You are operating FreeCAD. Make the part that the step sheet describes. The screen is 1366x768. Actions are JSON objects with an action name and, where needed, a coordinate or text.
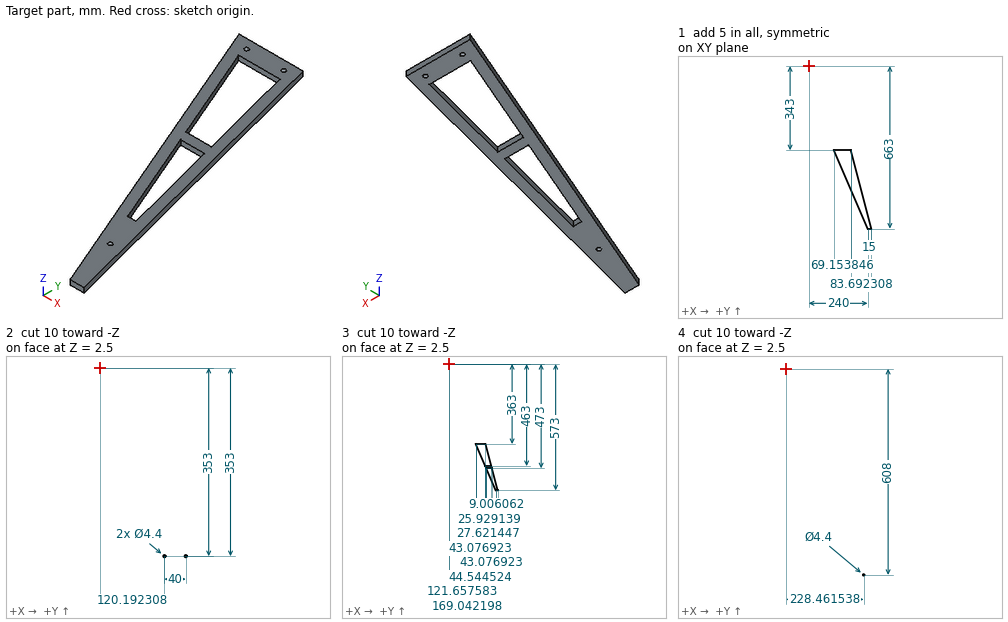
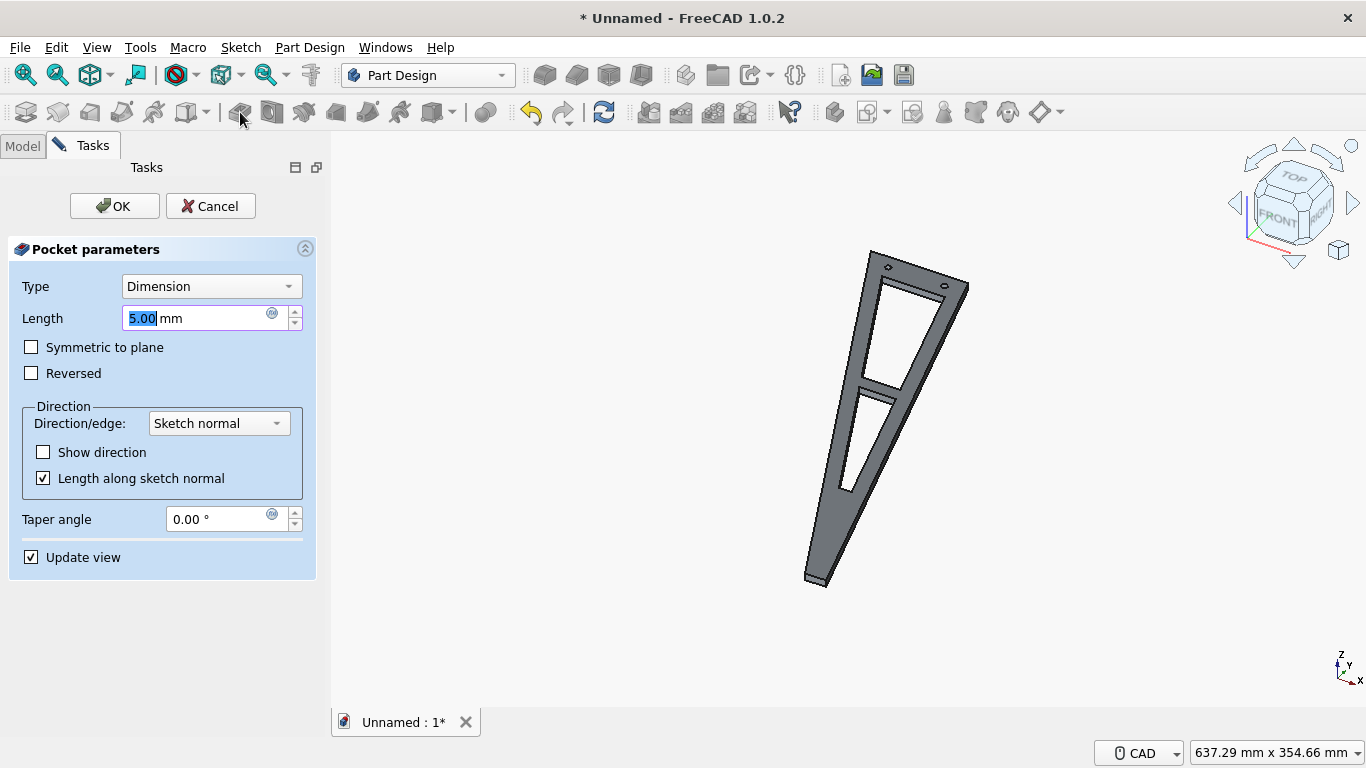
{"action": "type", "text": "10"}
{"action": "key", "text": "Tab"}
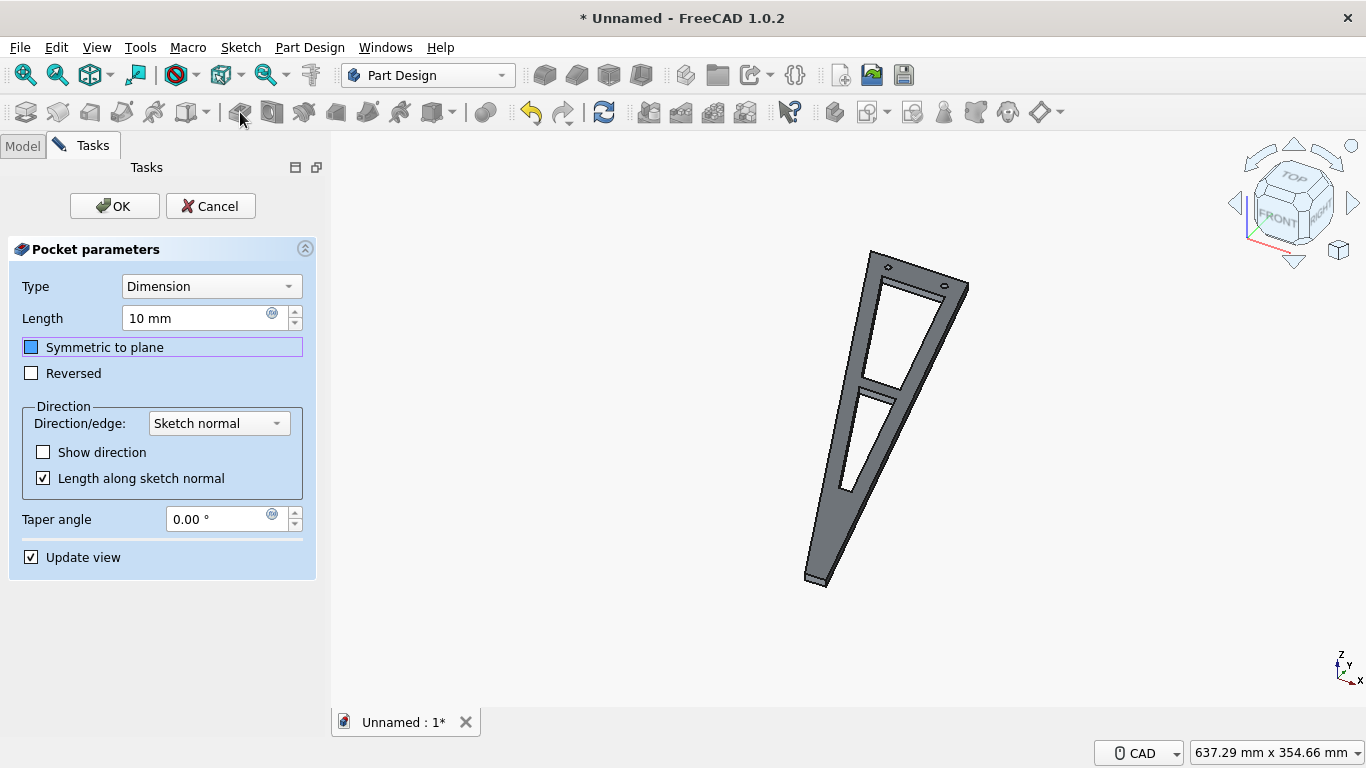
{"action": "left_click", "coordinate": [115, 206]}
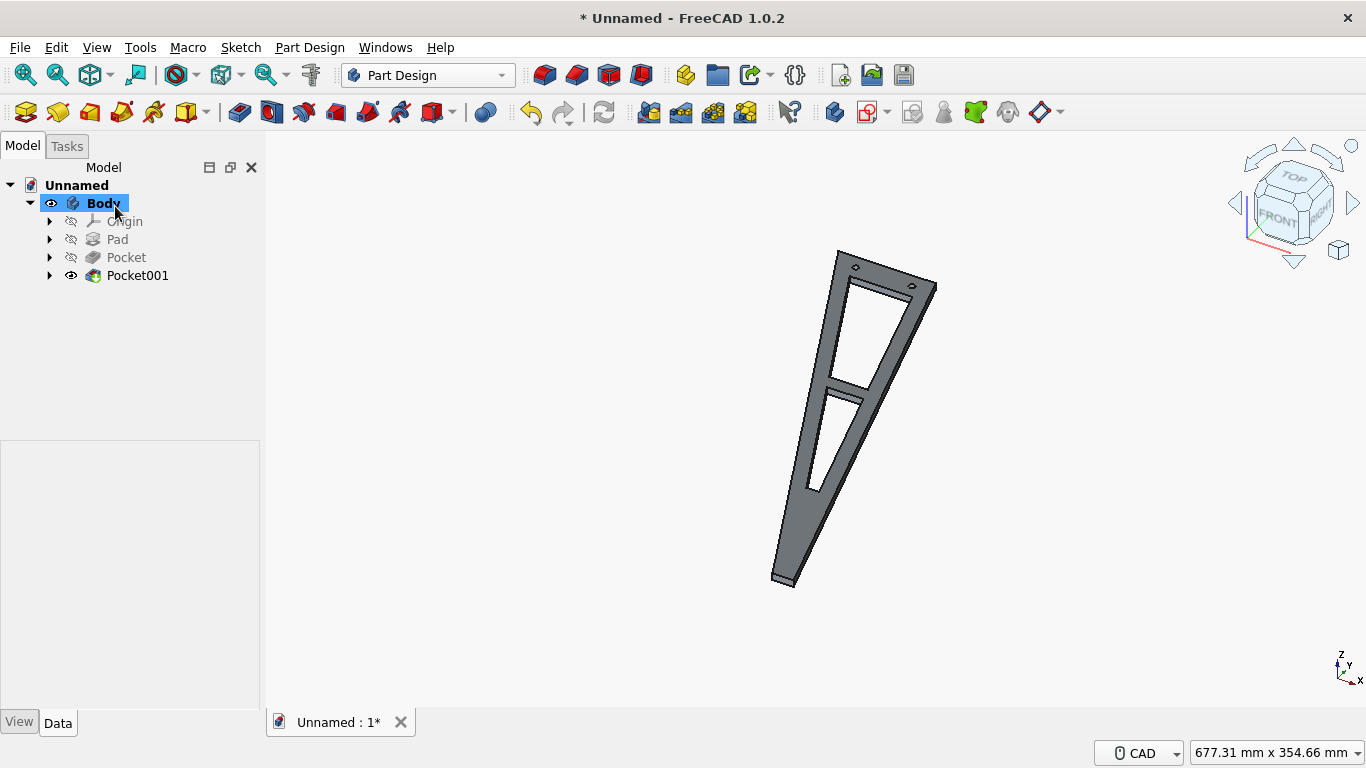
{"action": "left_click", "coordinate": [803, 509]}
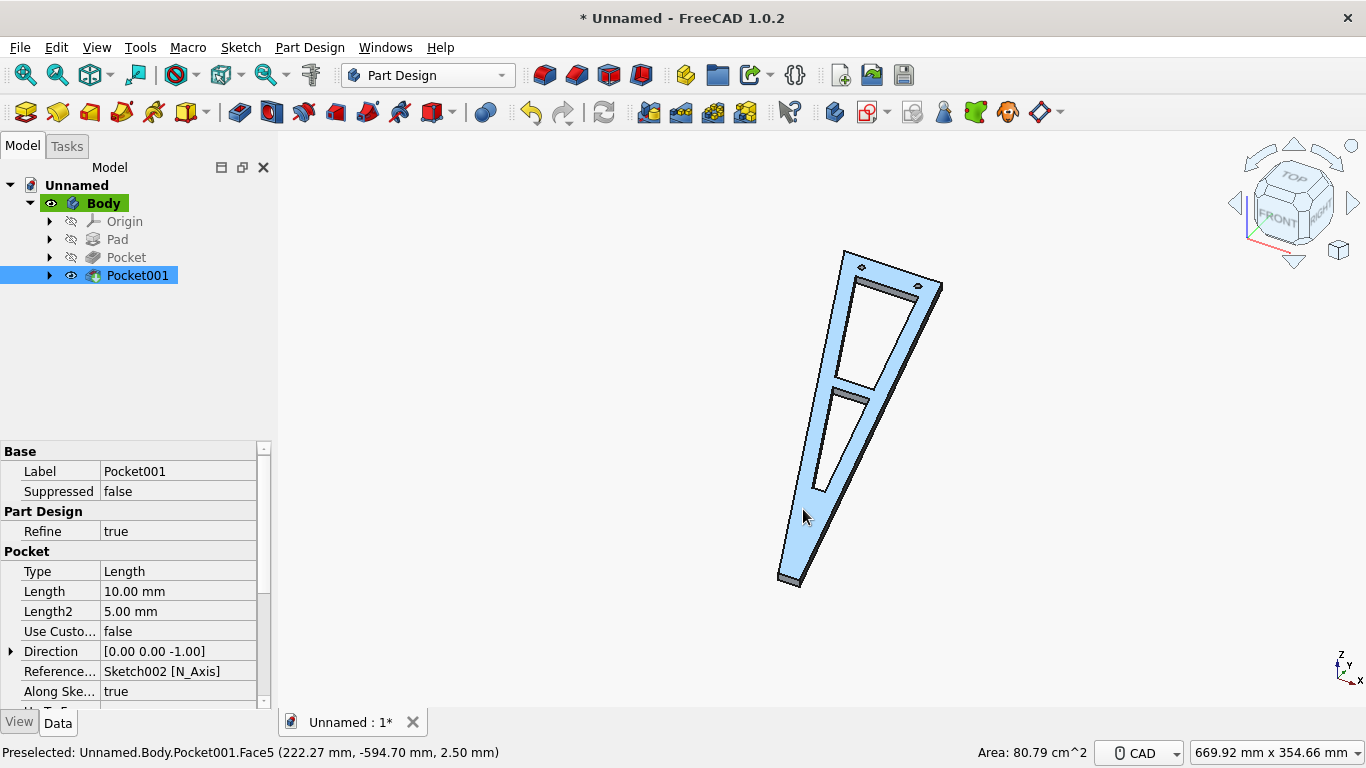
{"action": "left_click", "coordinate": [868, 112]}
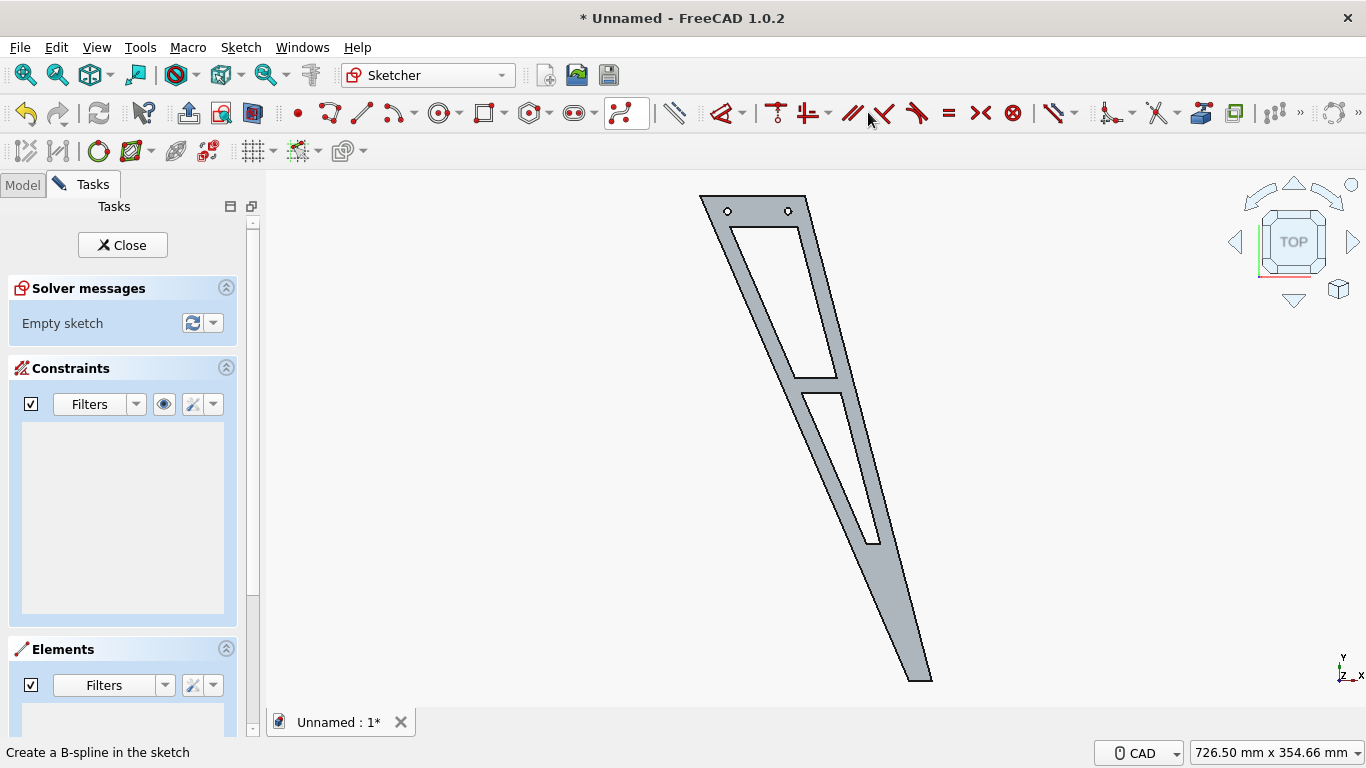
{"action": "scroll", "coordinate": [899, 606], "scroll_direction": "up", "scroll_amount": 15}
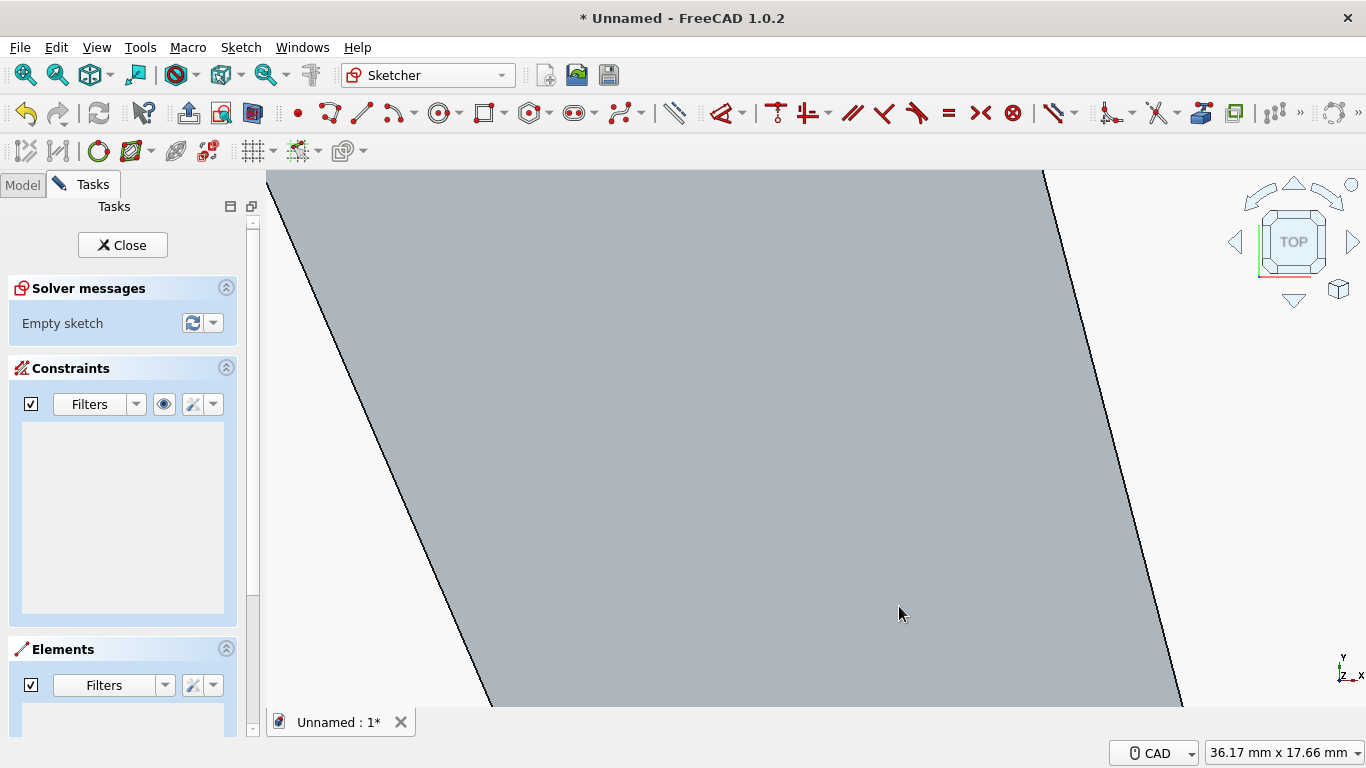
{"action": "scroll", "coordinate": [732, 408], "scroll_direction": "up", "scroll_amount": 5}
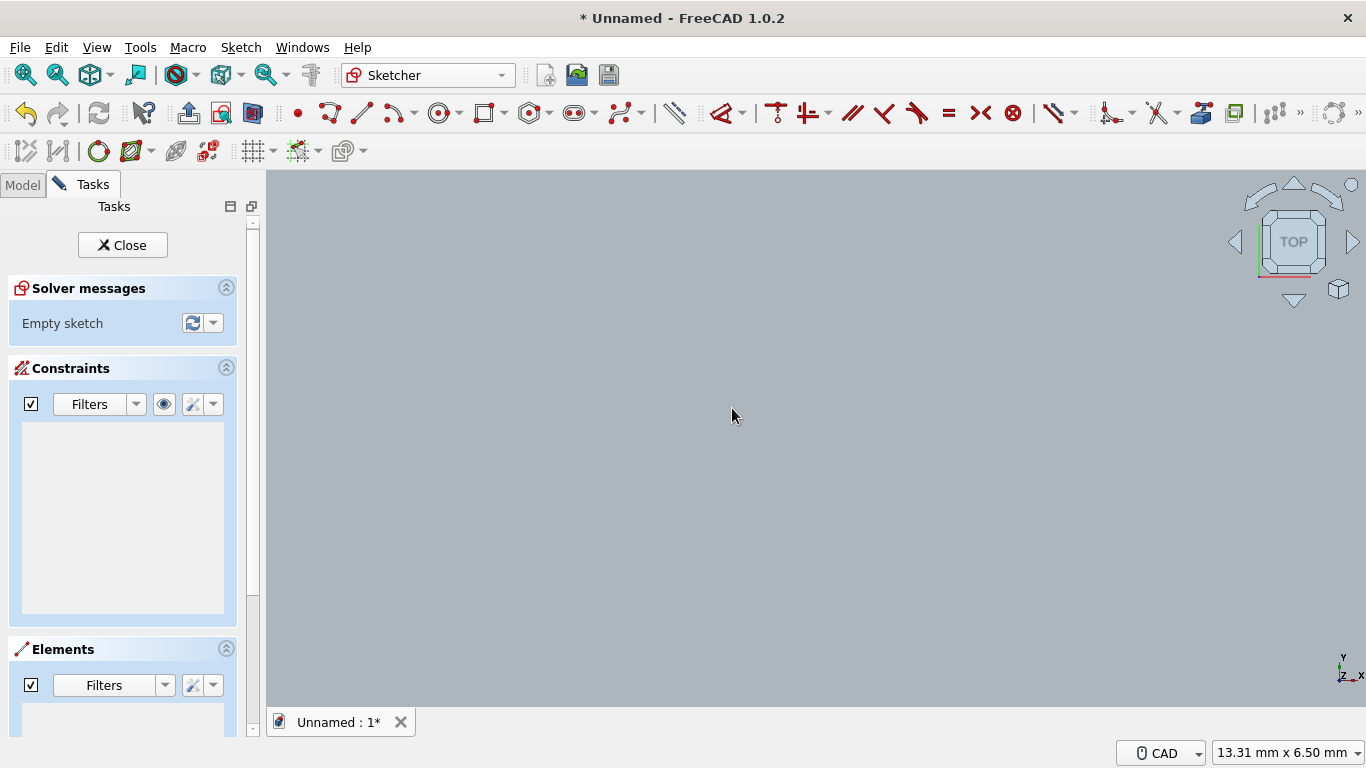
{"action": "left_click", "coordinate": [440, 114]}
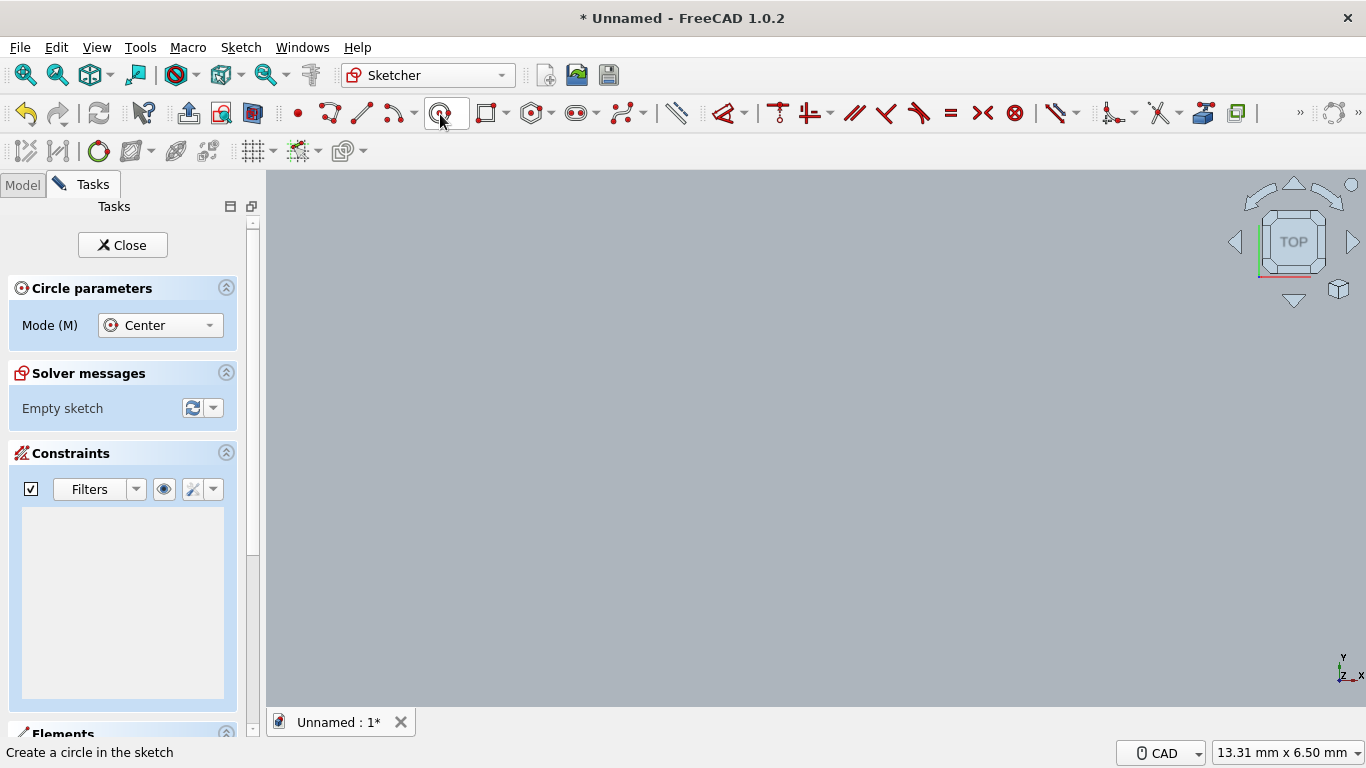
{"action": "left_click", "coordinate": [748, 438]}
{"action": "mouse_move", "coordinate": [876, 310]}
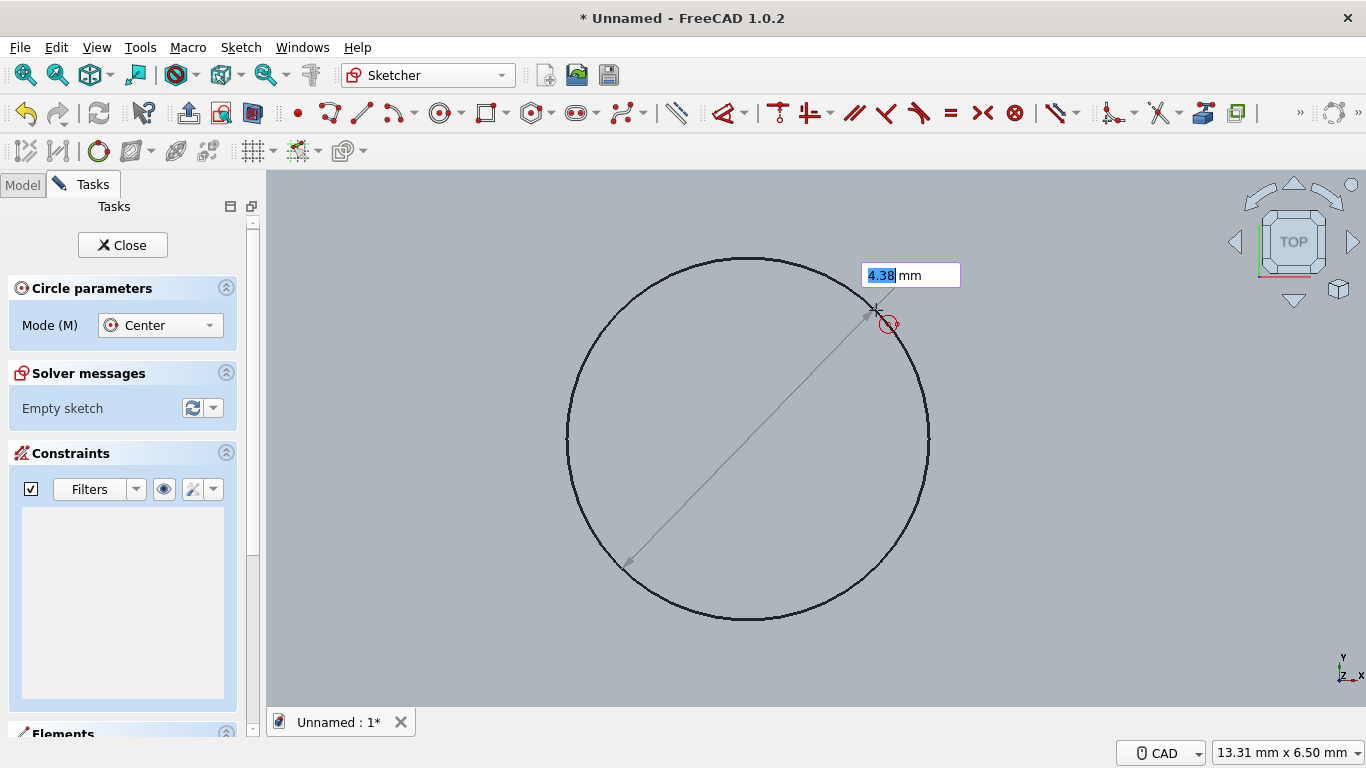
{"action": "type", "text": "4.4"}
{"action": "key", "text": "Return"}
{"action": "key", "text": "Escape"}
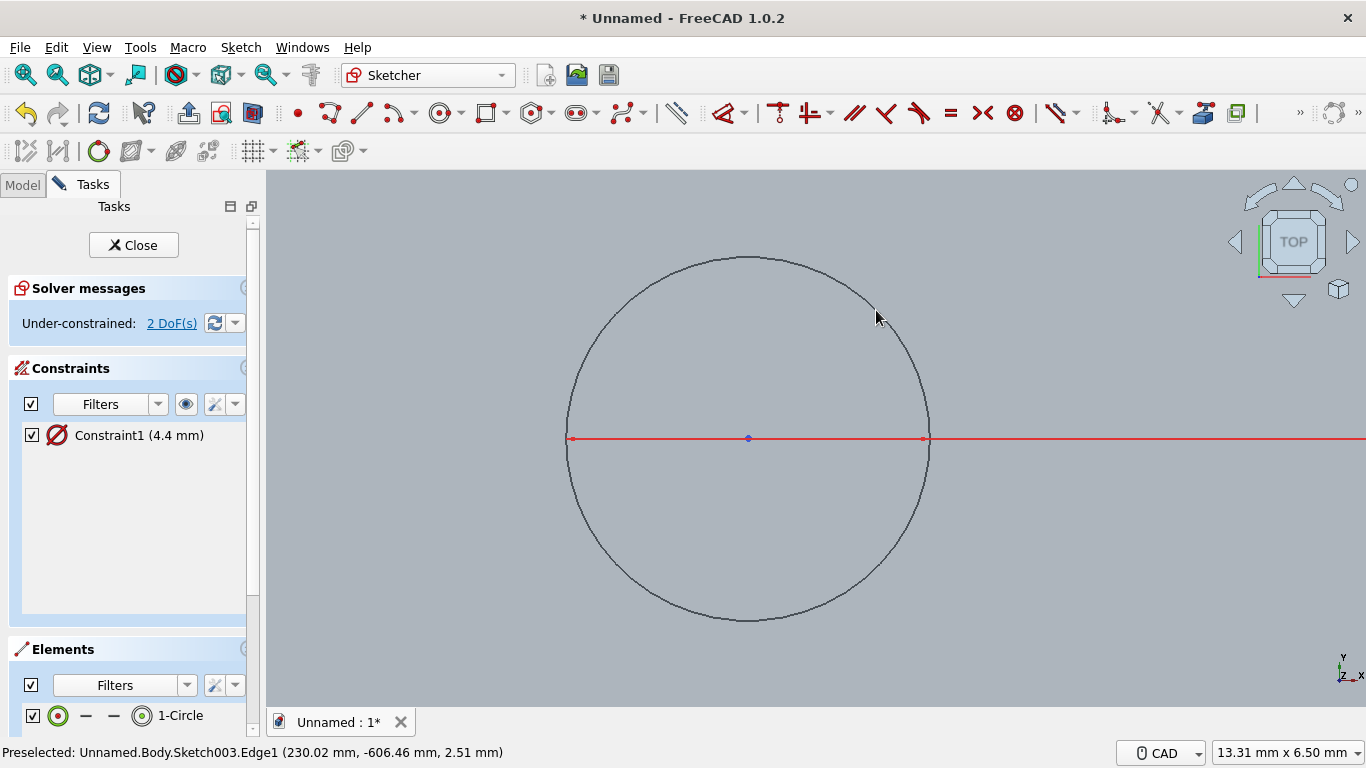
{"action": "left_click", "coordinate": [724, 114]}